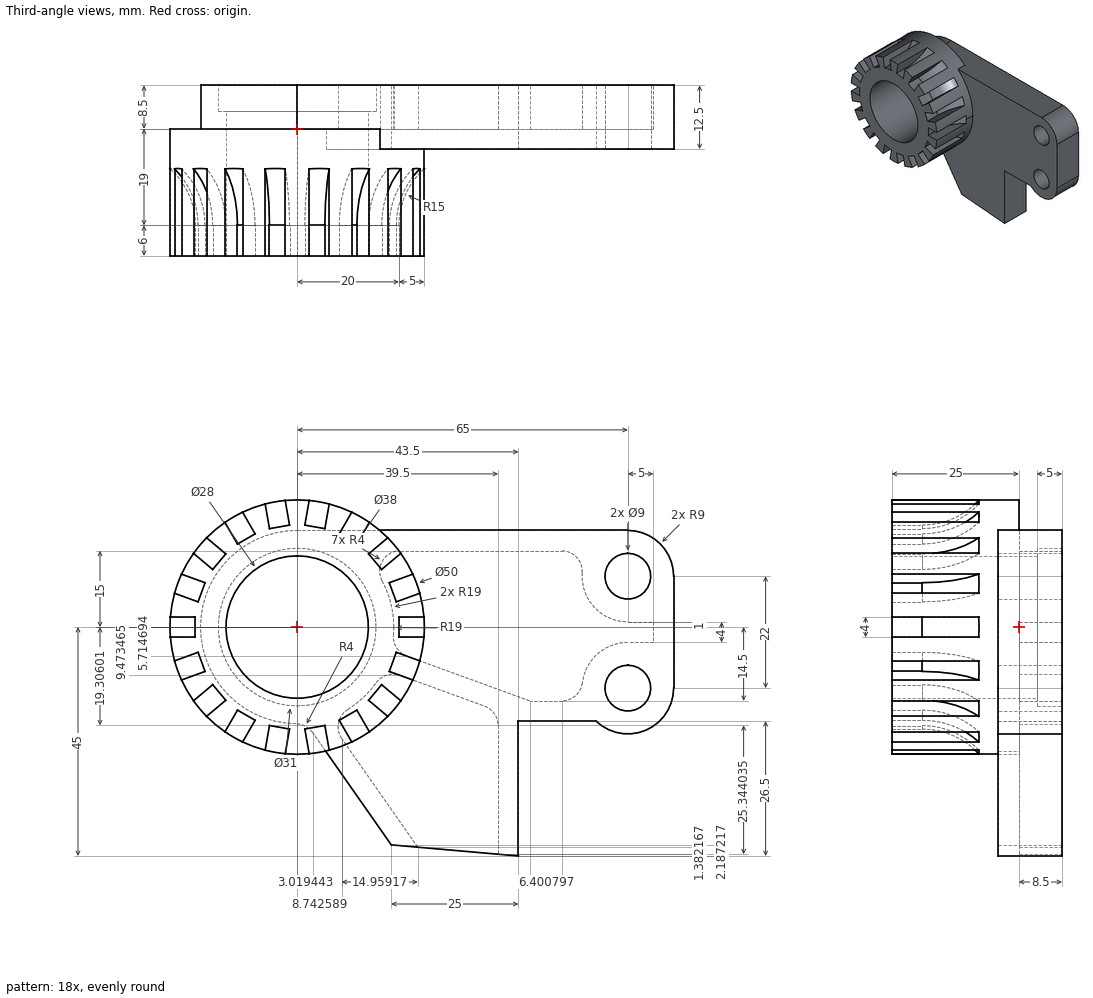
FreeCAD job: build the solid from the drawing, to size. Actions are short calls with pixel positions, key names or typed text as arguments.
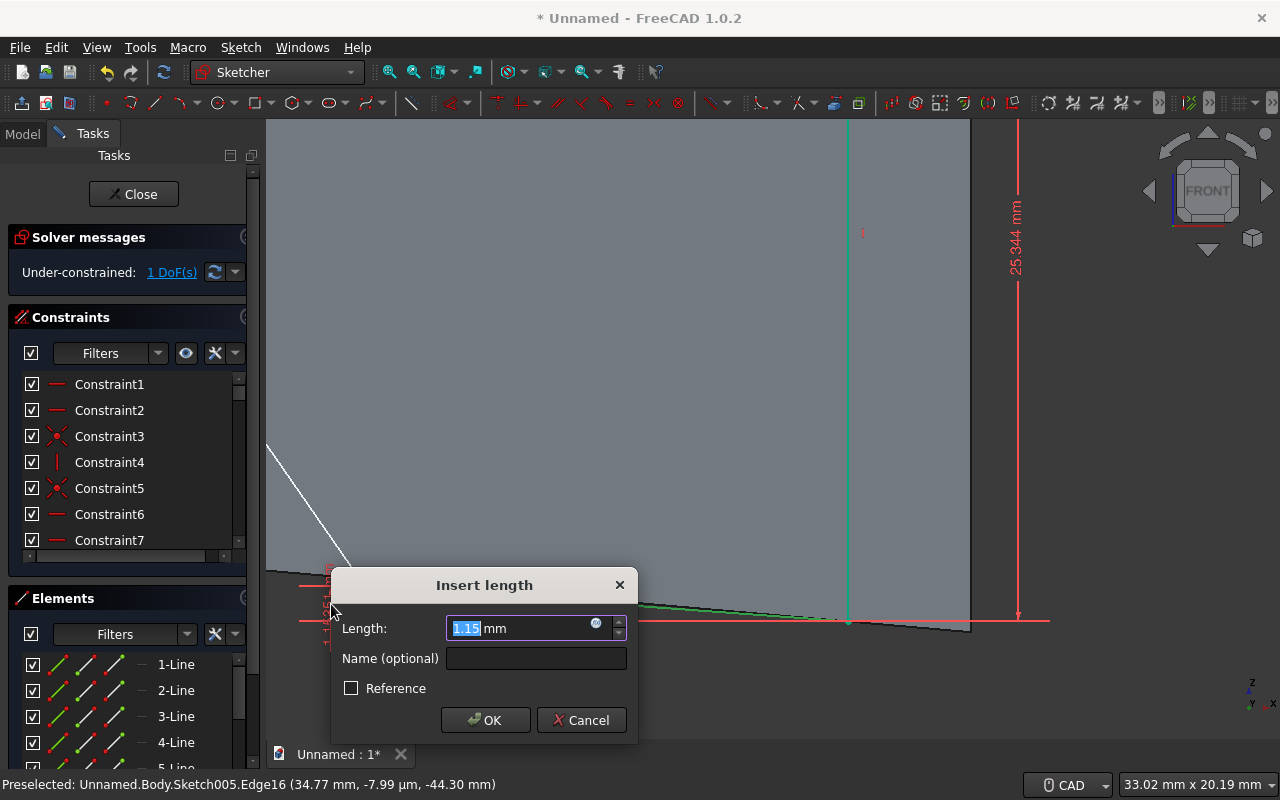
text(1.382167)
key(Return)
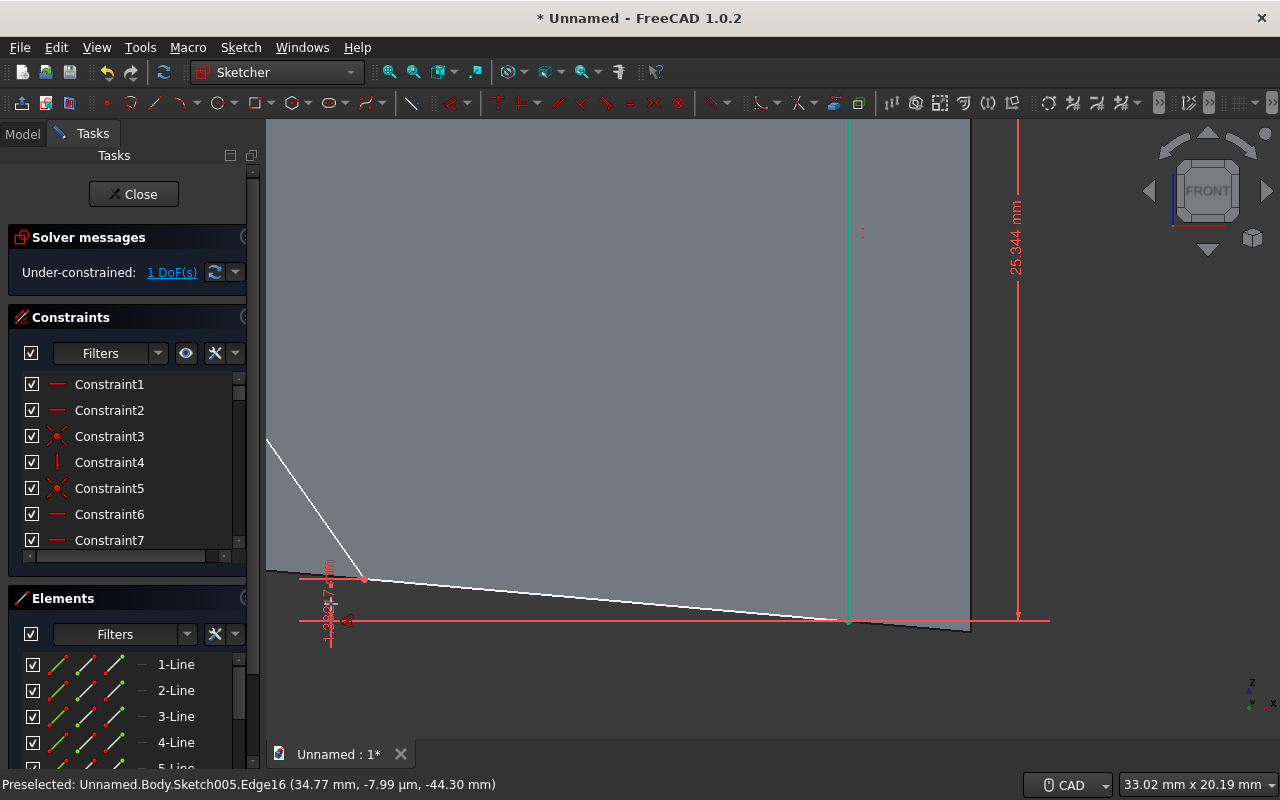
scroll(703, 612, down, 8)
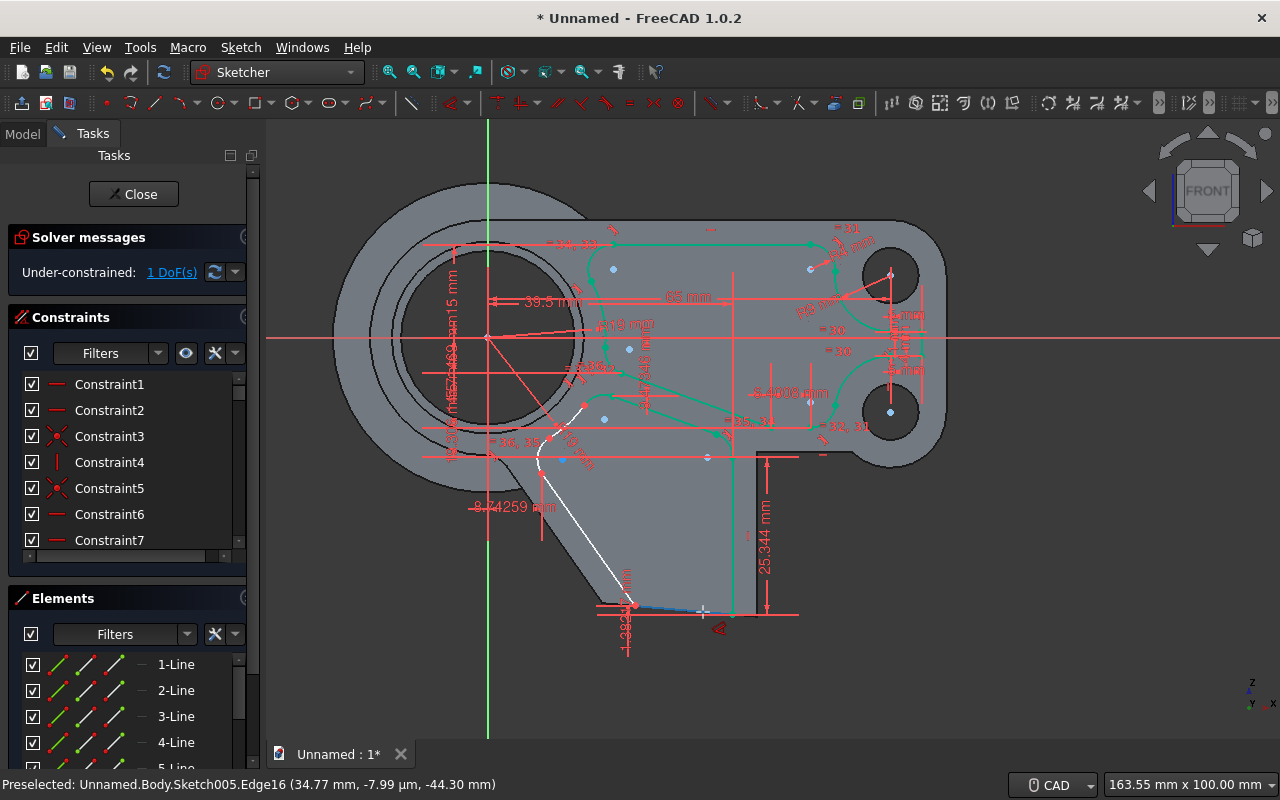
click(607, 566)
click(589, 640)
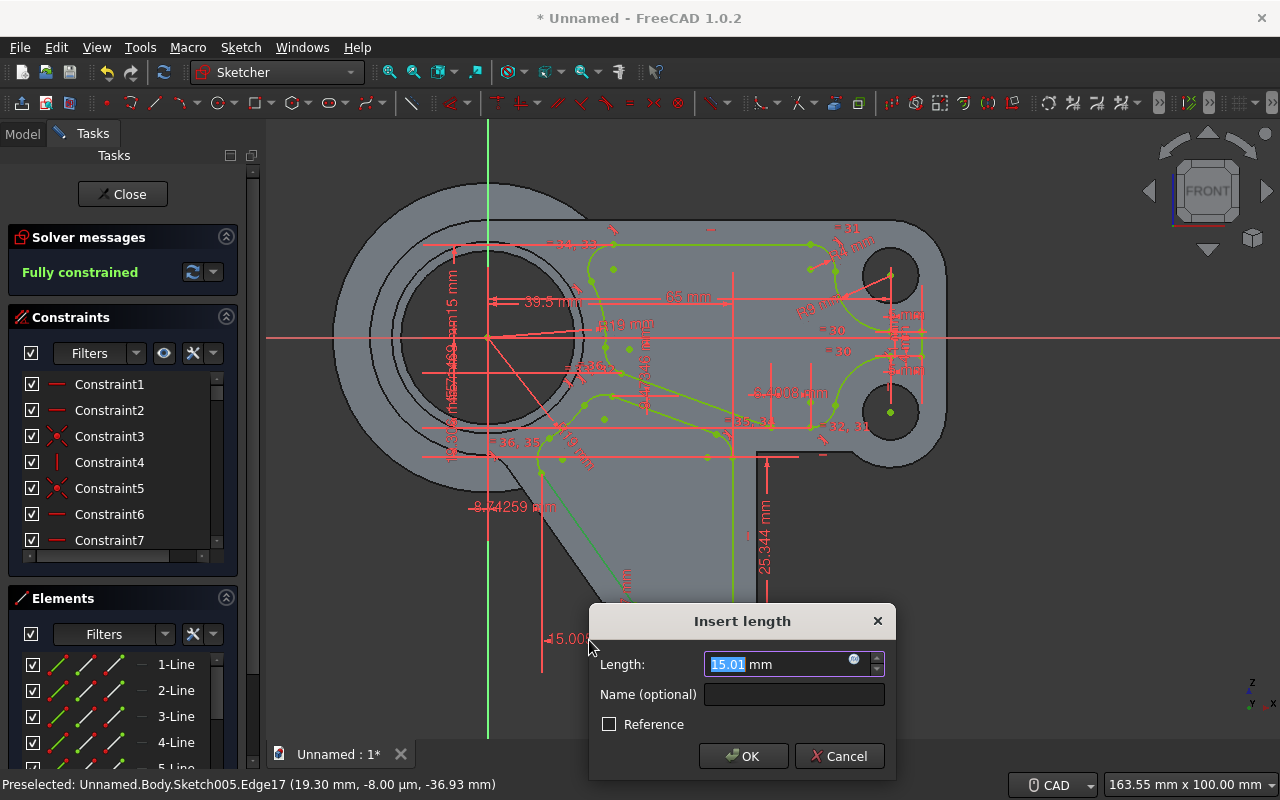
text(14.95917)
key(Return)
key(Escape)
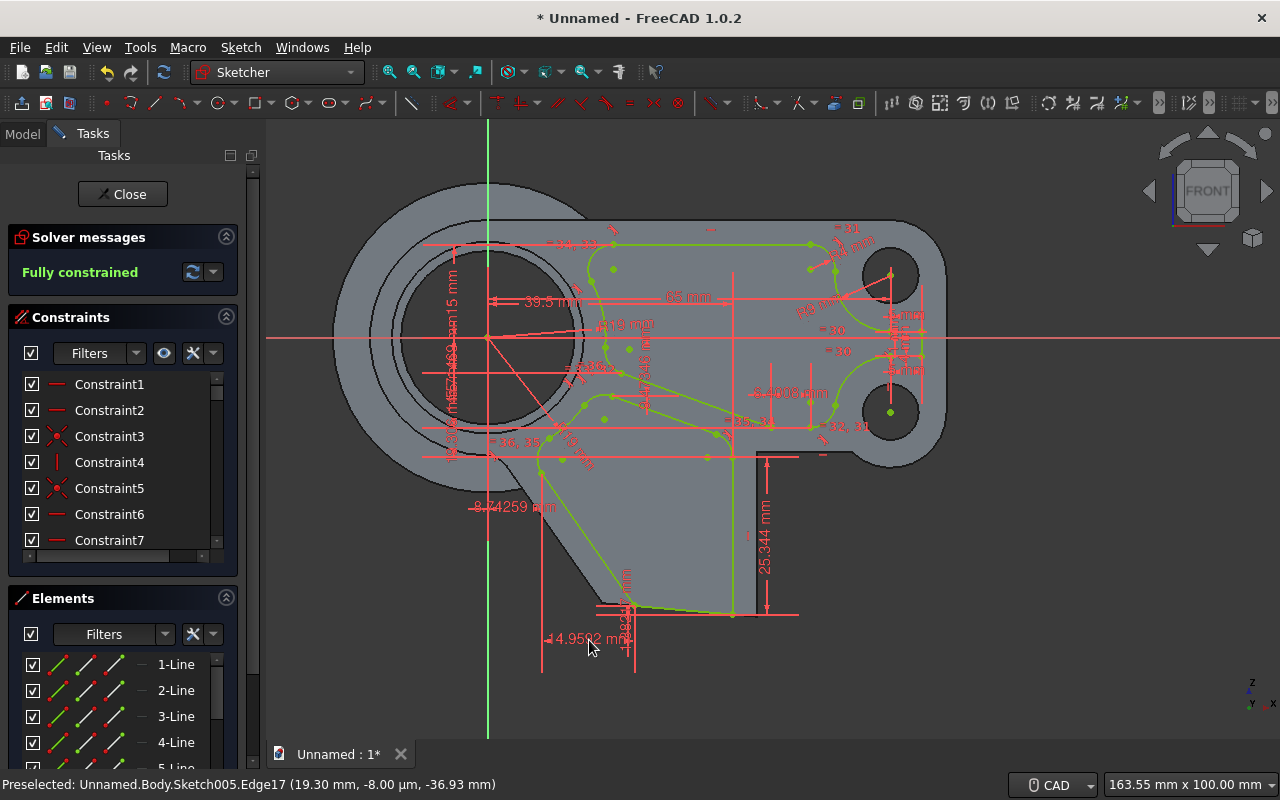
click(123, 194)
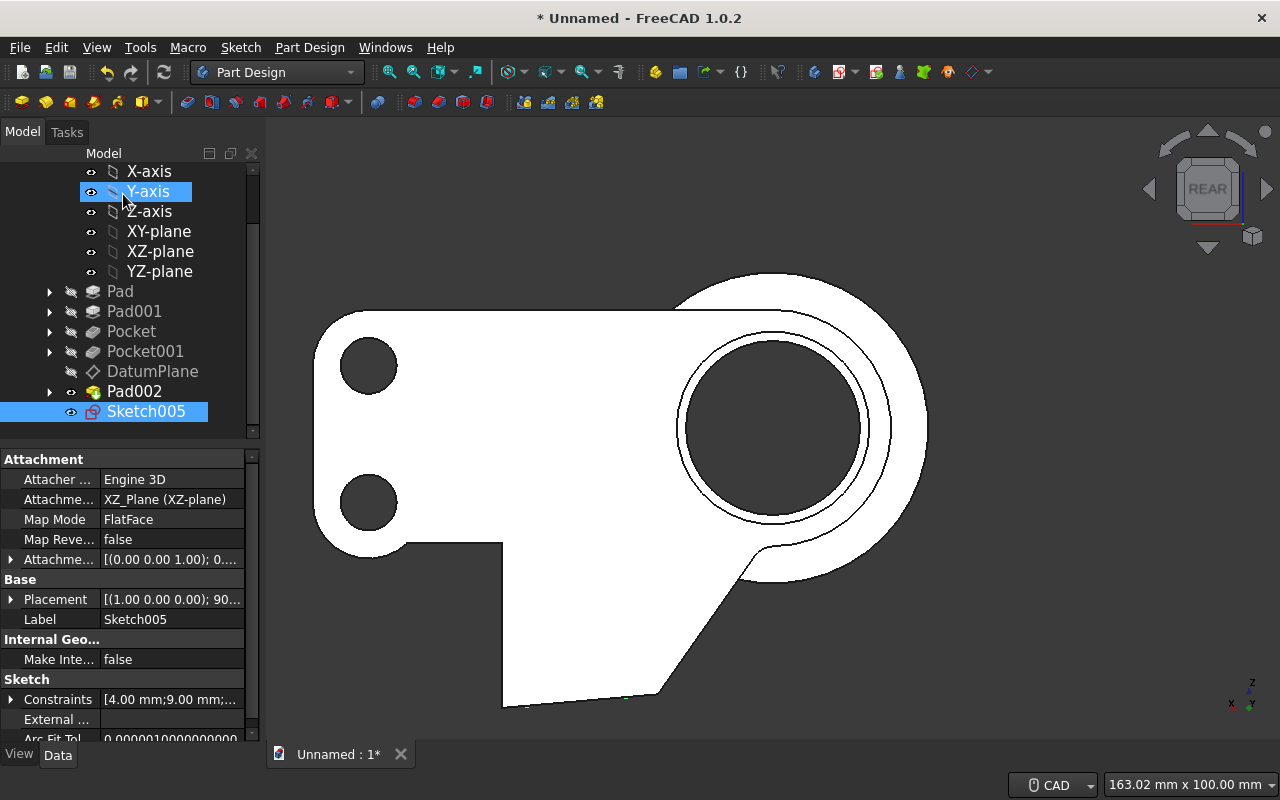
click(188, 102)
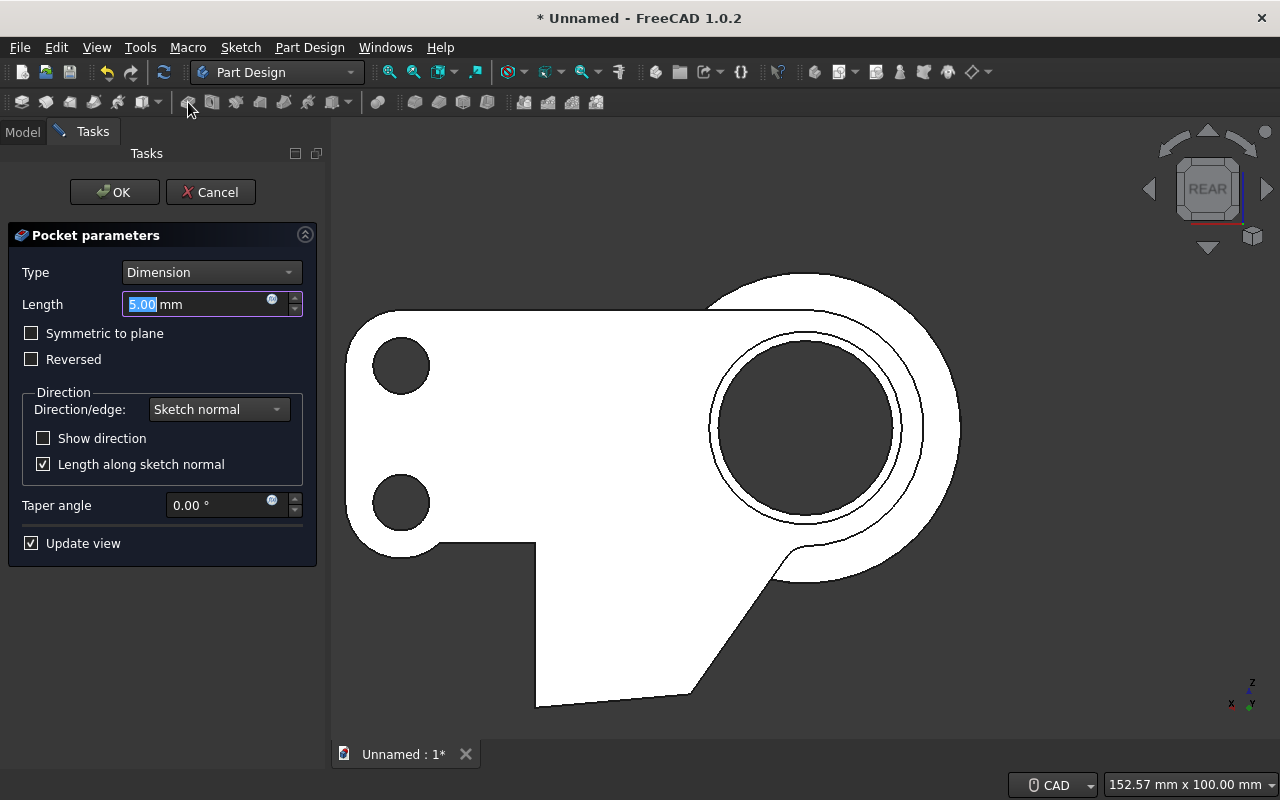
text(8.5)
key(Tab)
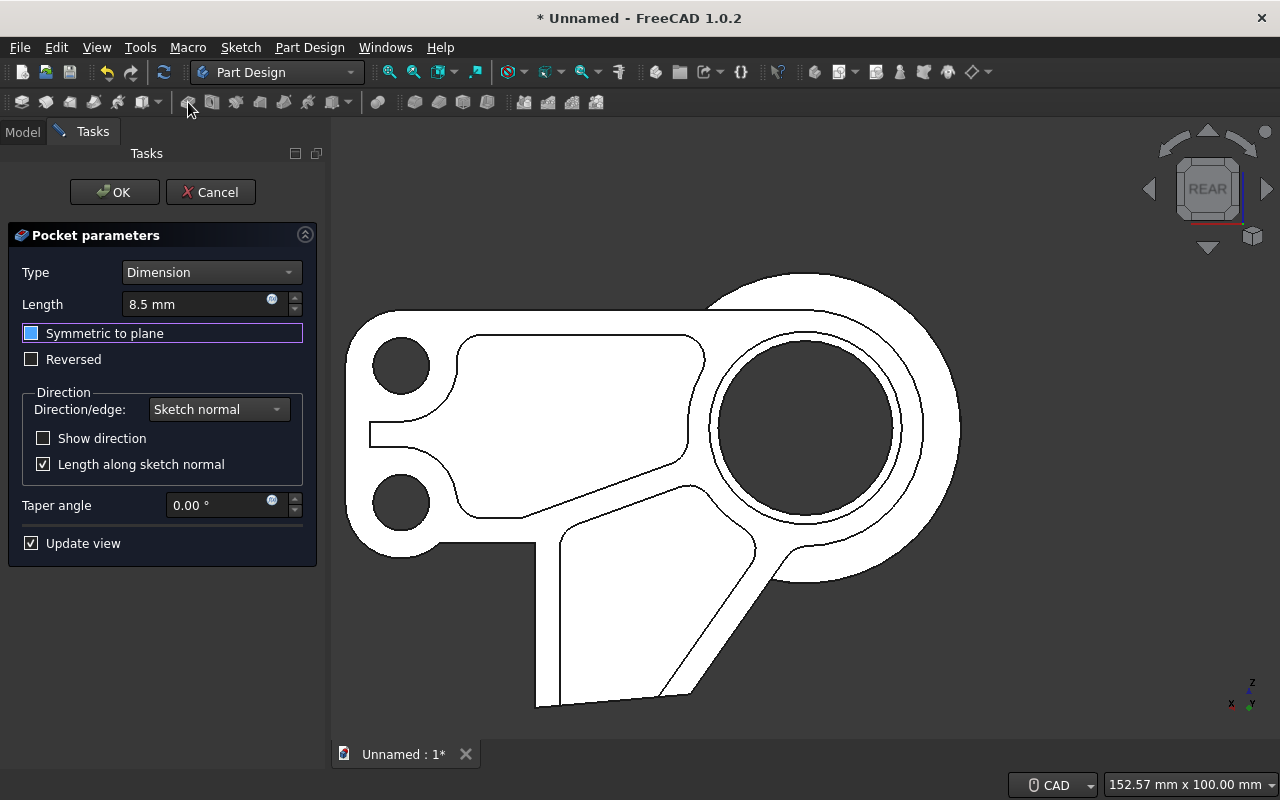
click(115, 192)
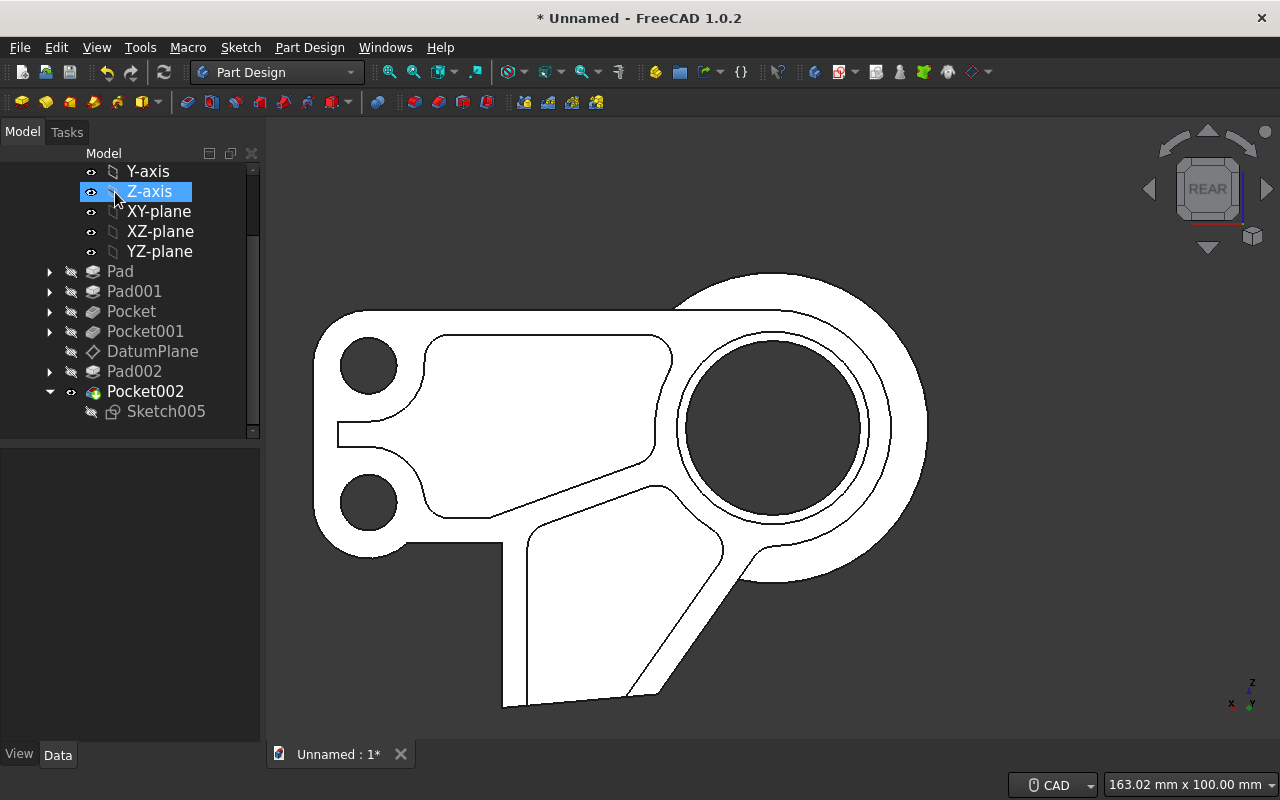
click(840, 72)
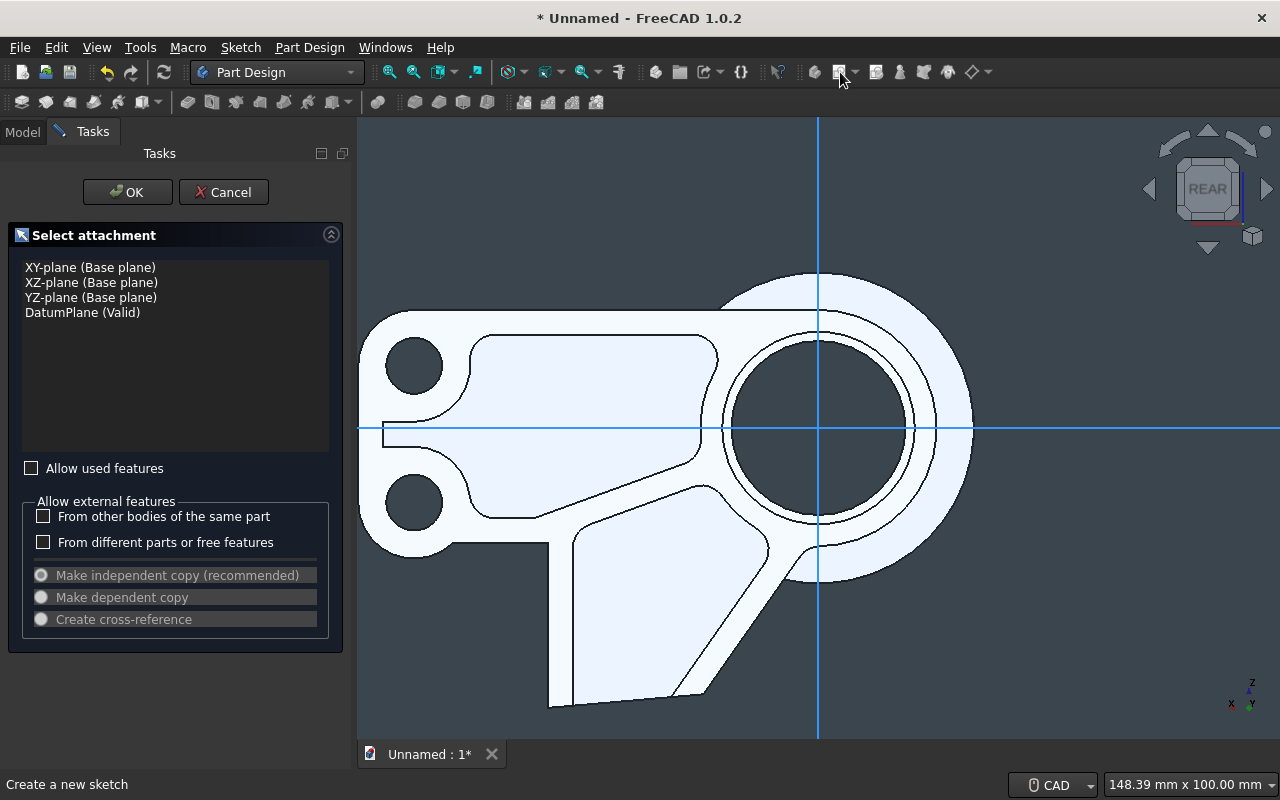
click(82, 268)